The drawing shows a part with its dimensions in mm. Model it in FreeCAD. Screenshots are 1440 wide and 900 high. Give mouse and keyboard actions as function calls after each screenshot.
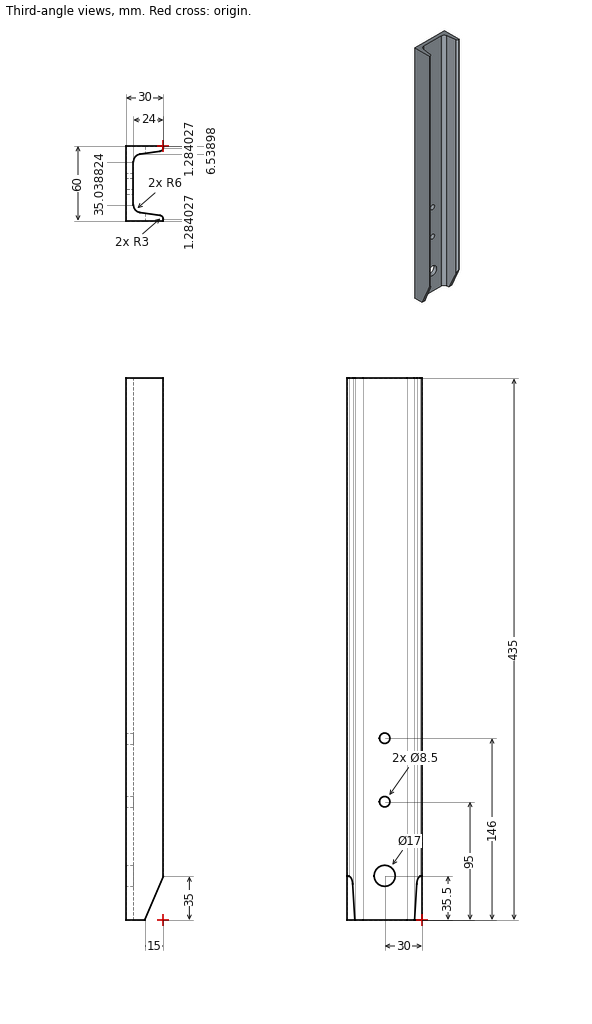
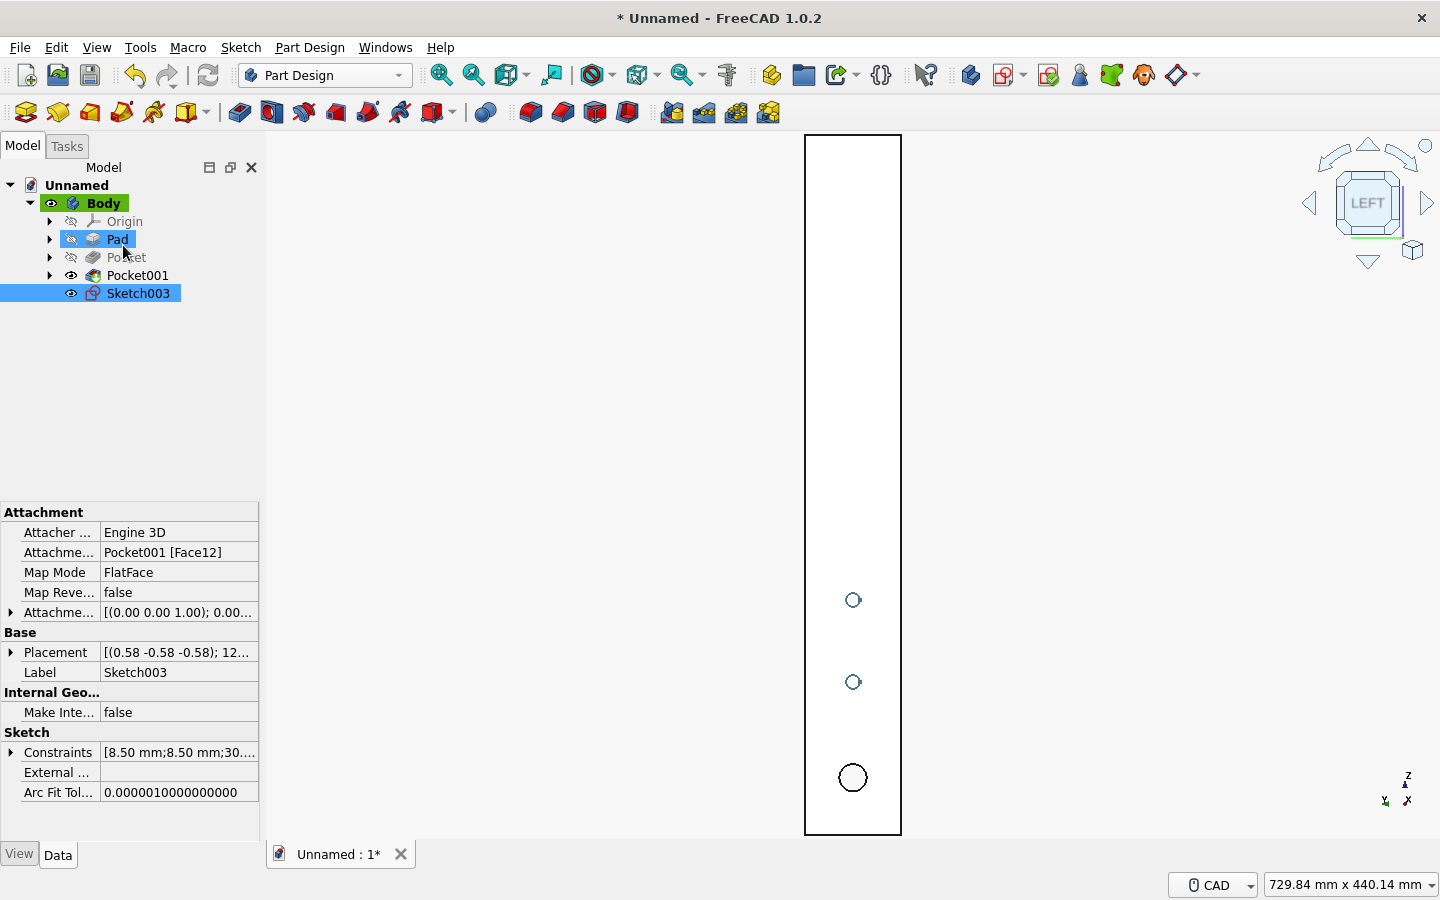
click(240, 112)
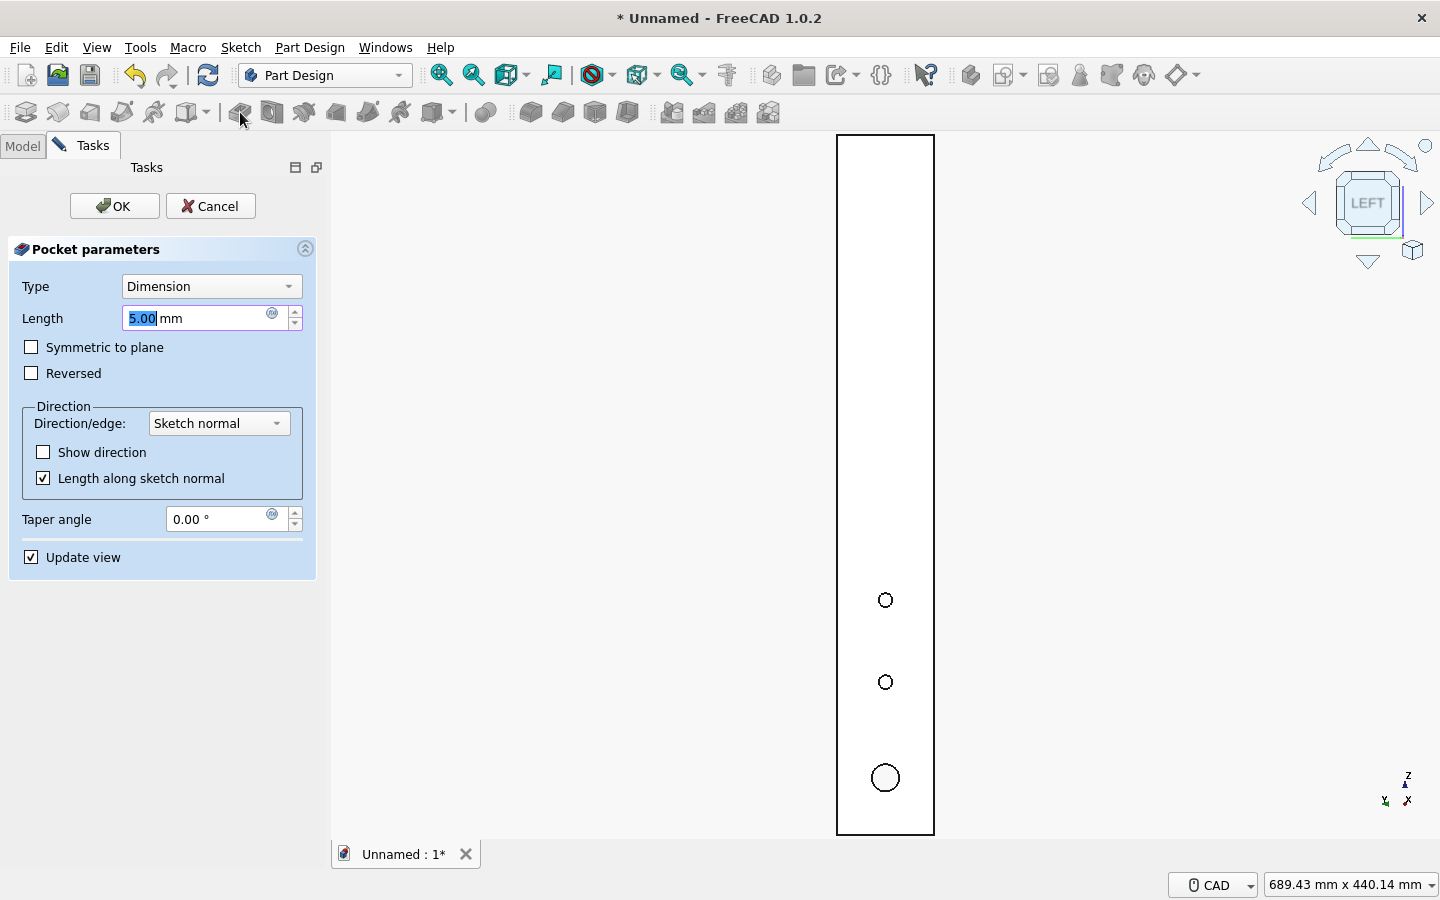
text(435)
key(Tab)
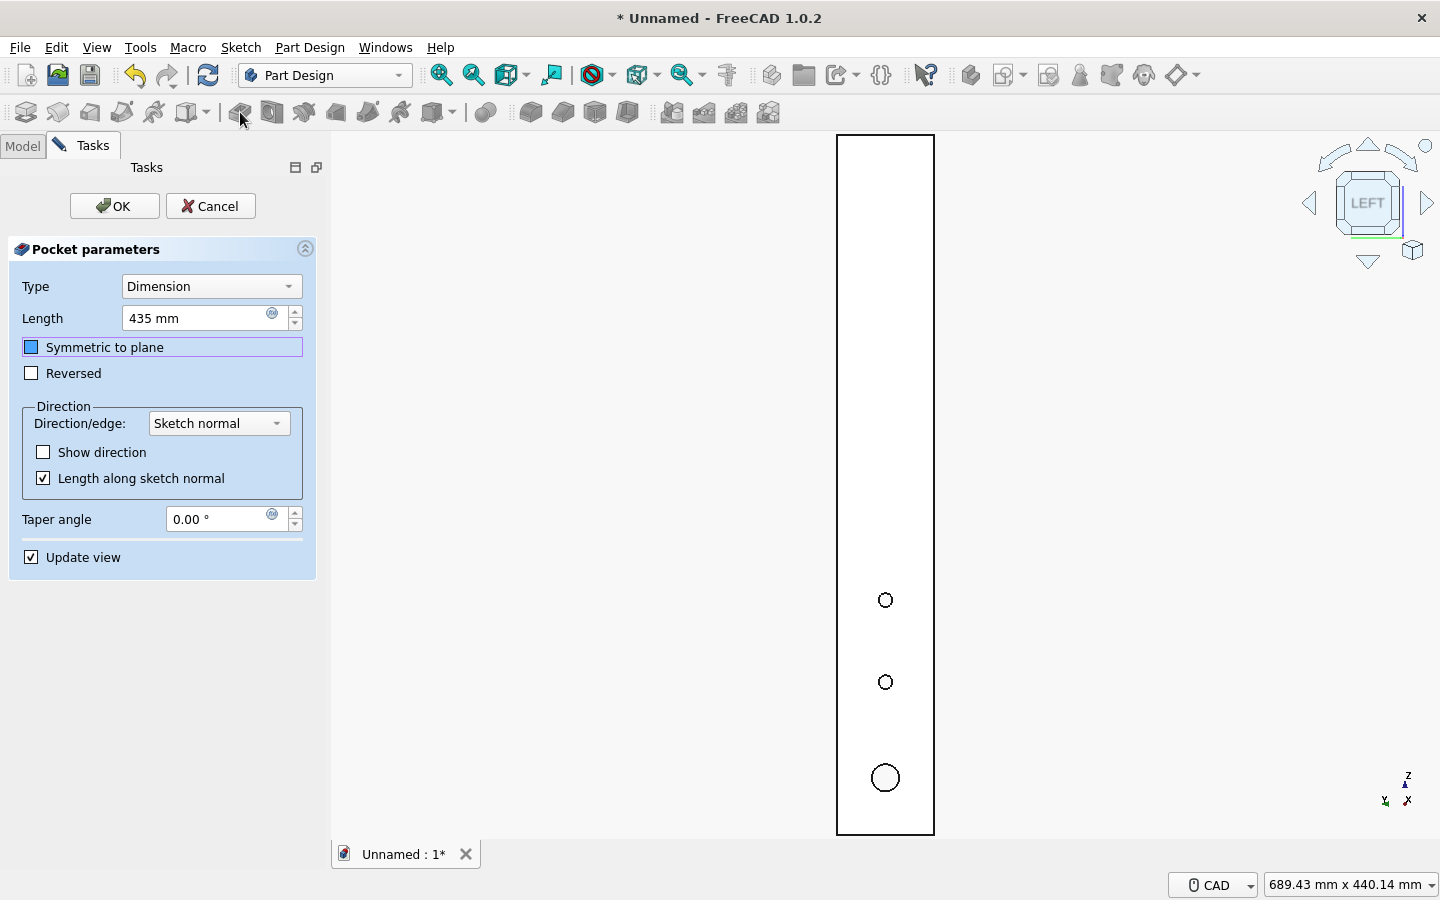
click(115, 206)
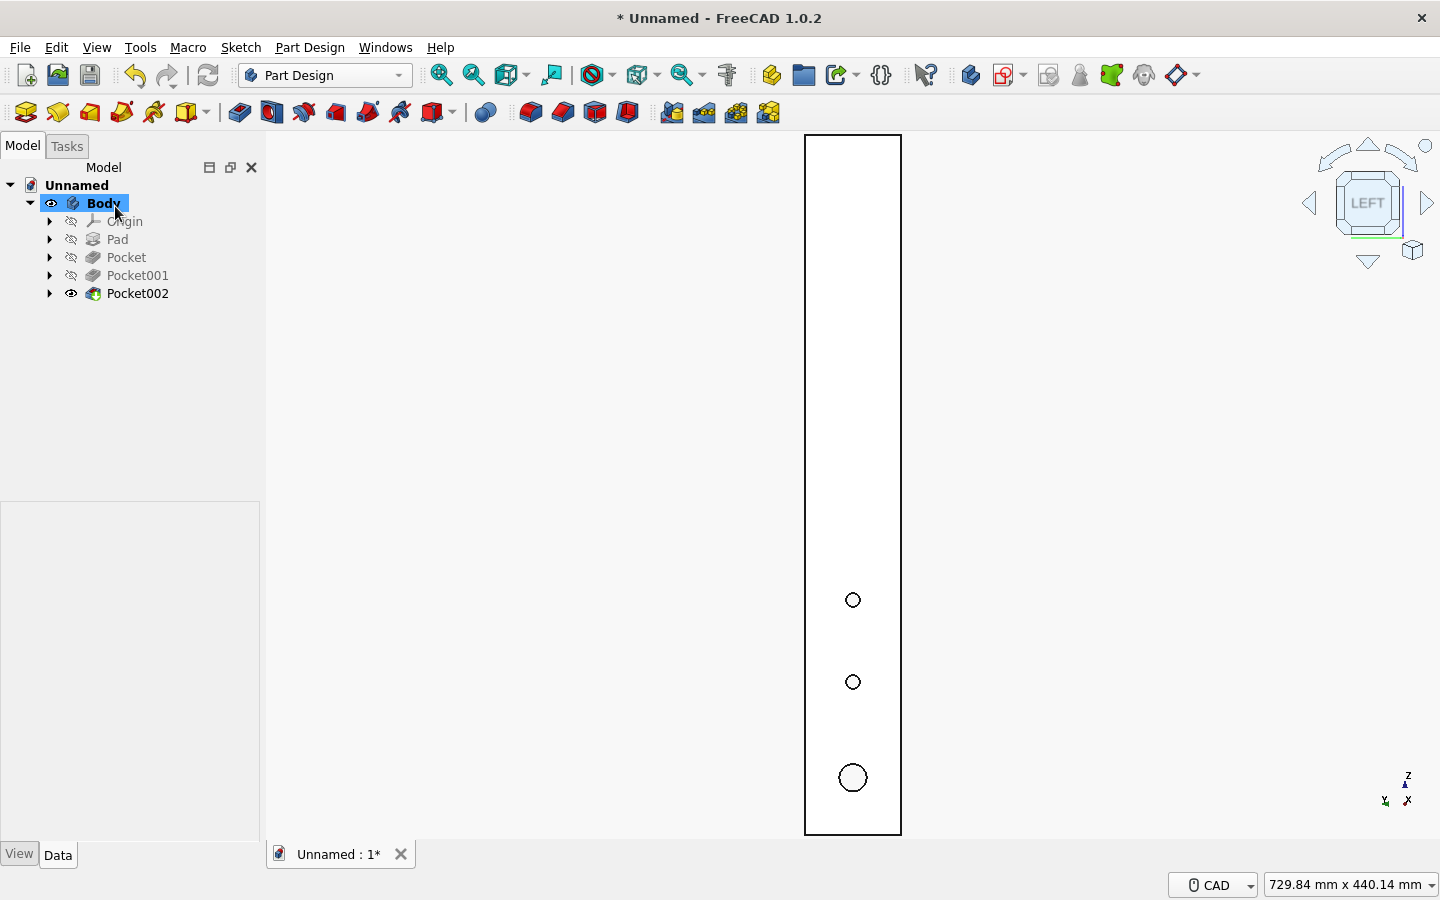
key(0)